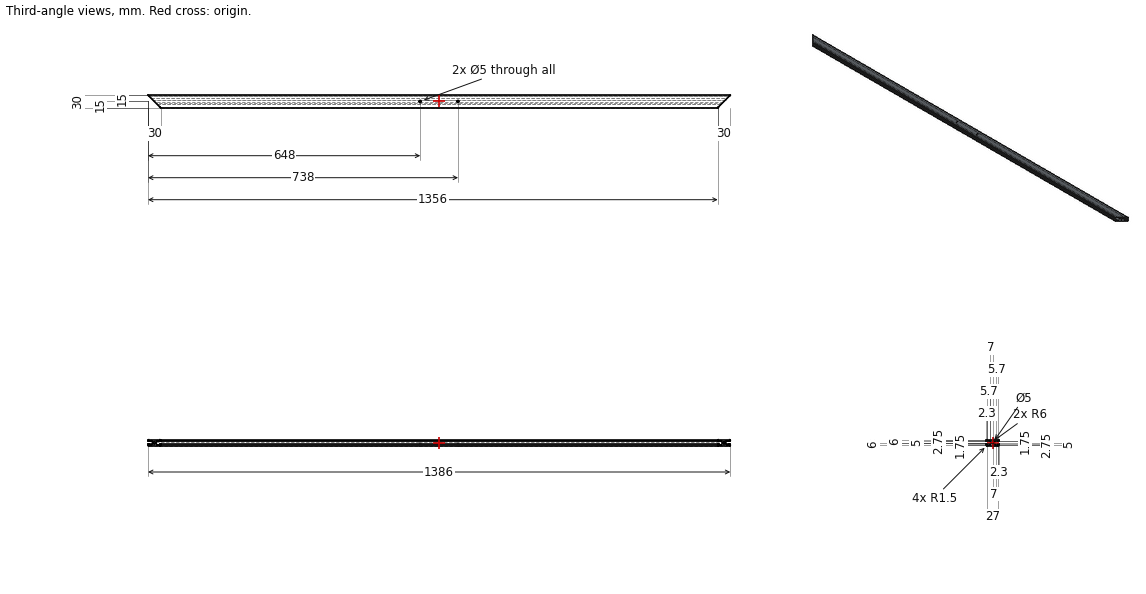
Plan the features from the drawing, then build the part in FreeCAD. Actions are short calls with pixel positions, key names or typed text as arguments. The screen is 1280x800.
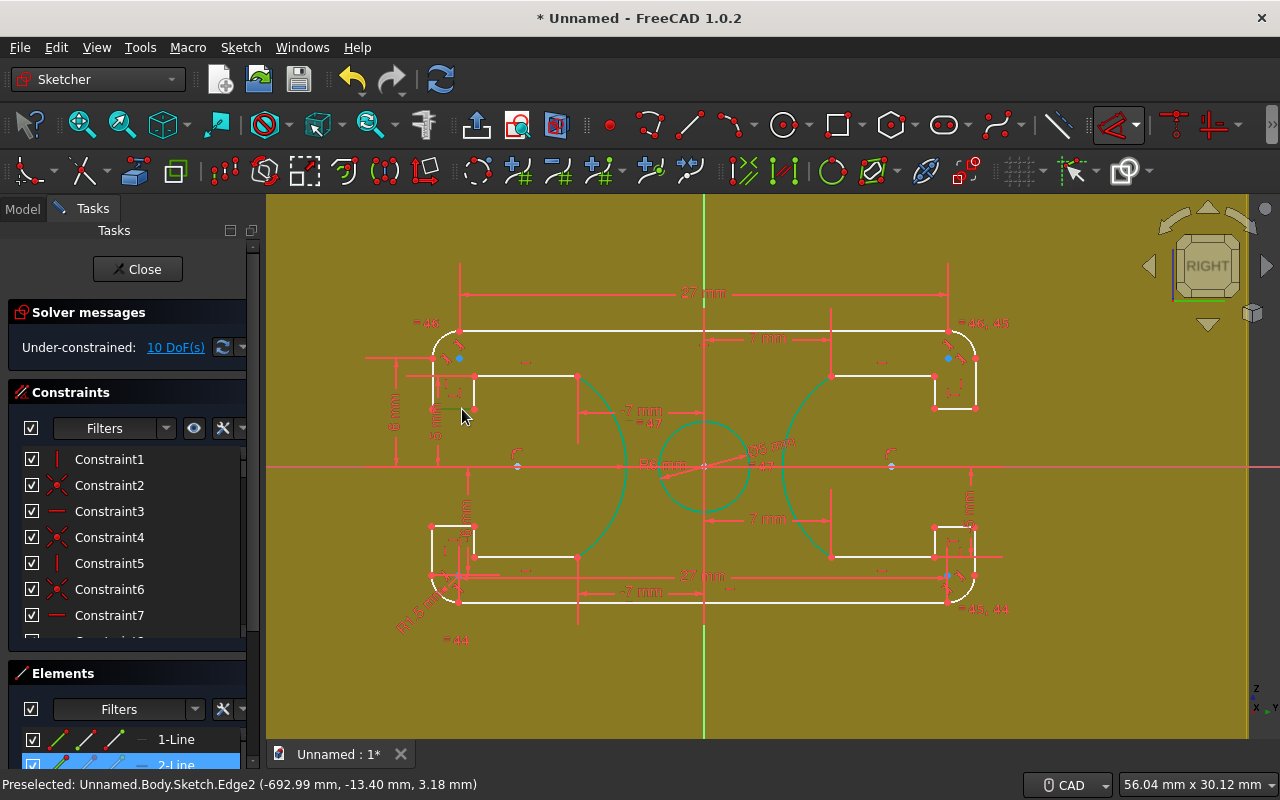
click(1138, 126)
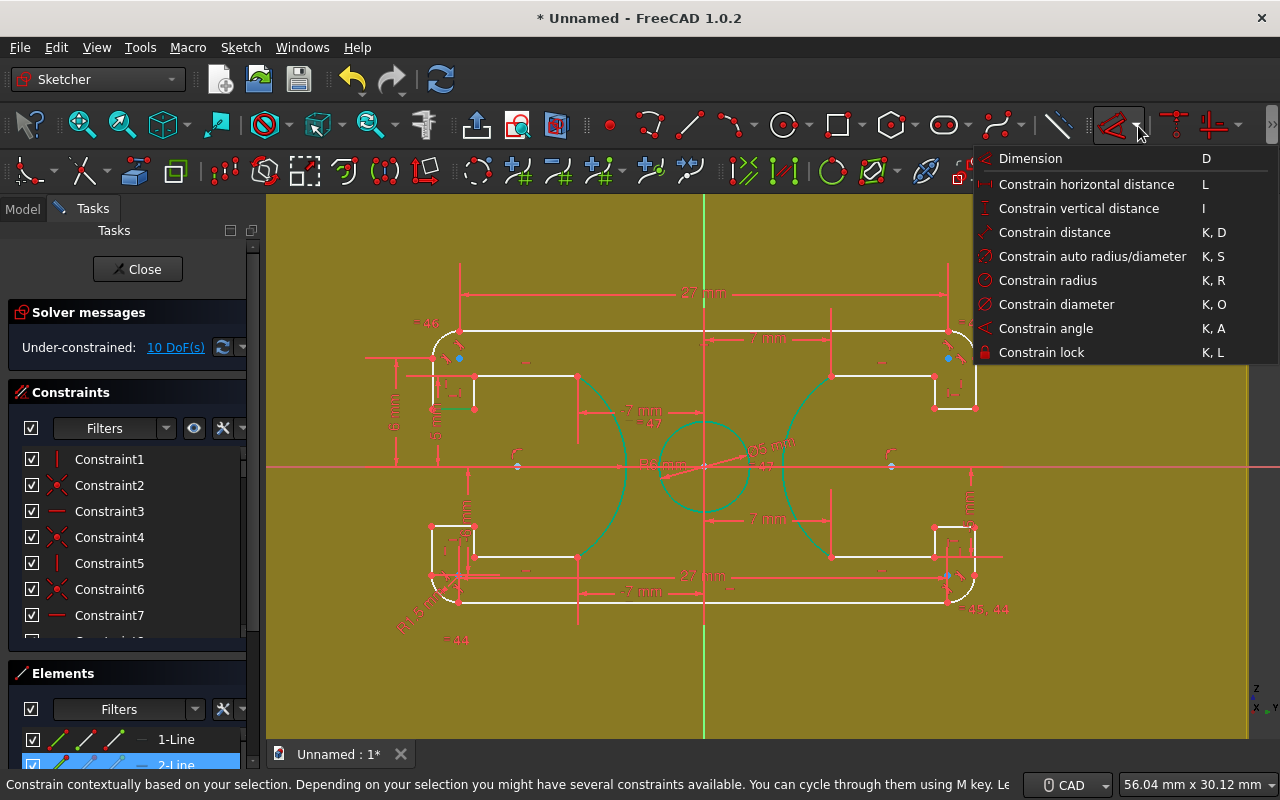
click(1126, 184)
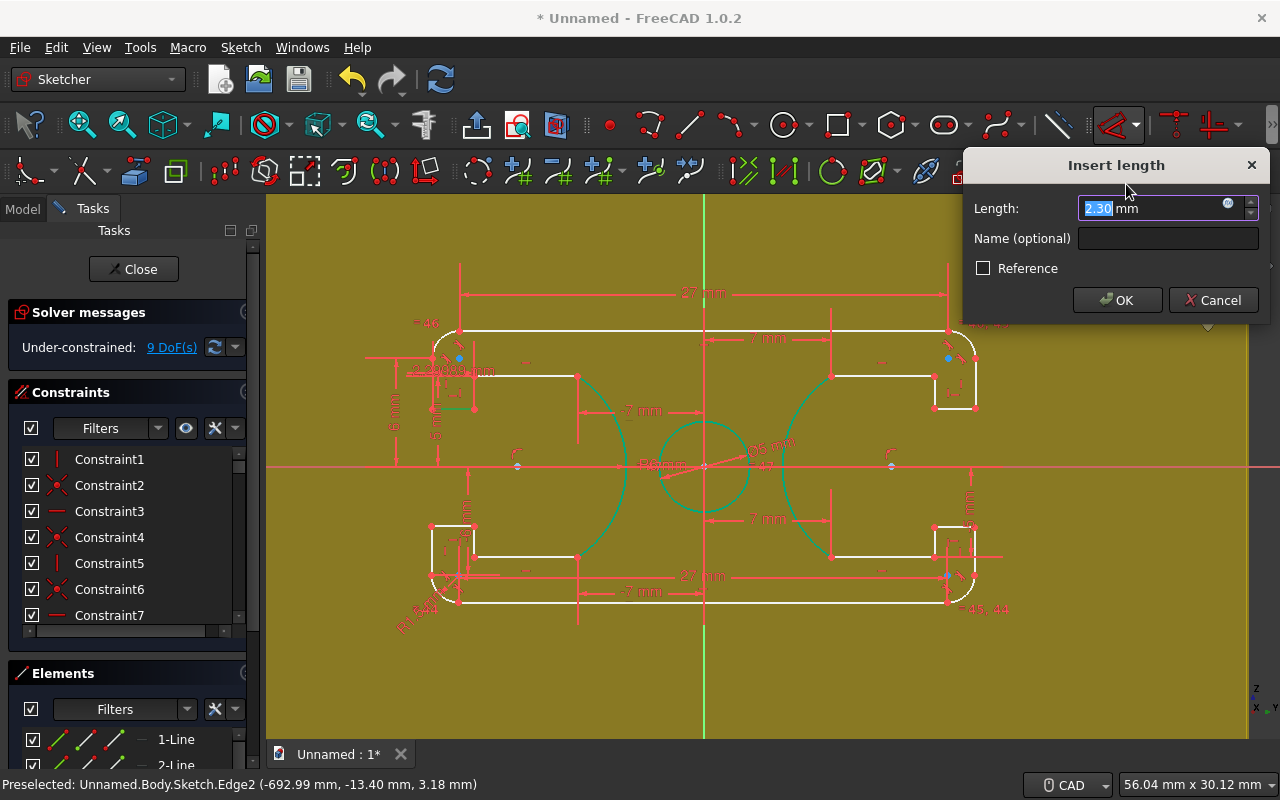
text(2.3)
key(Return)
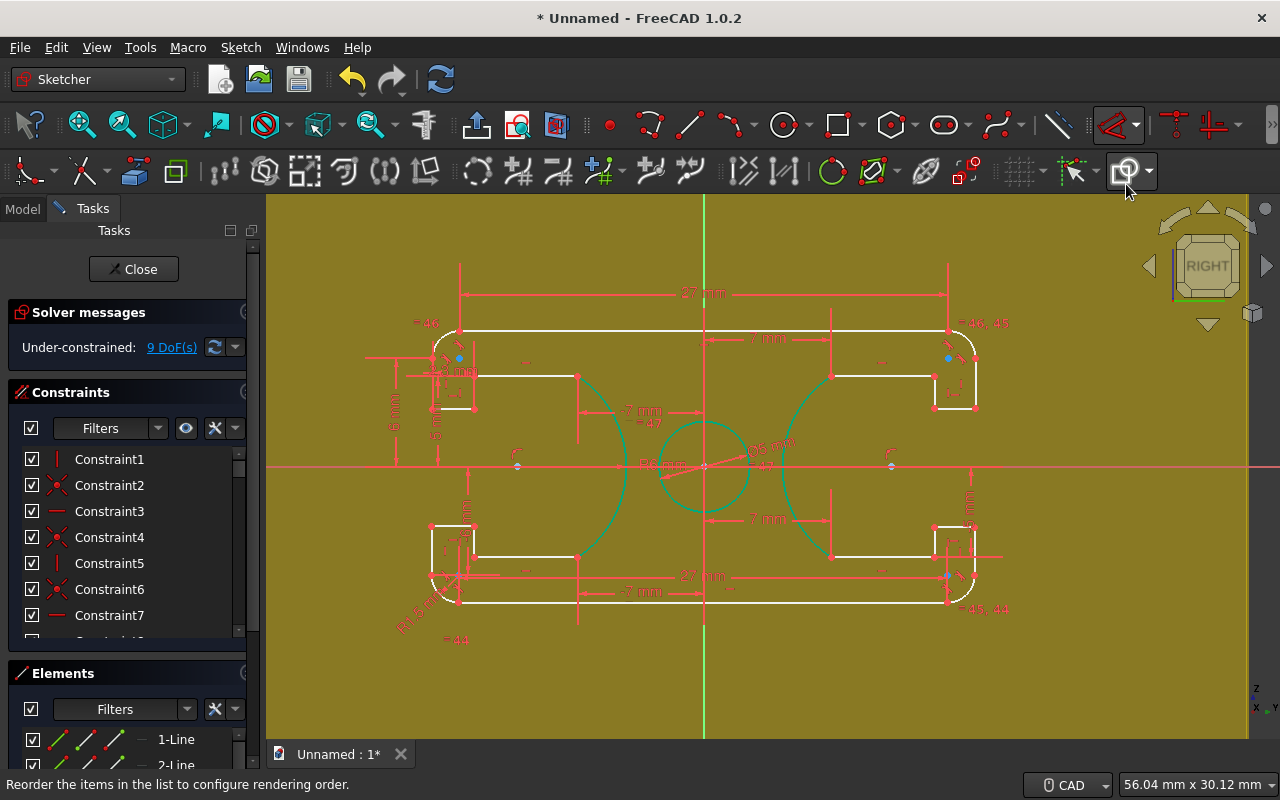
click(505, 376)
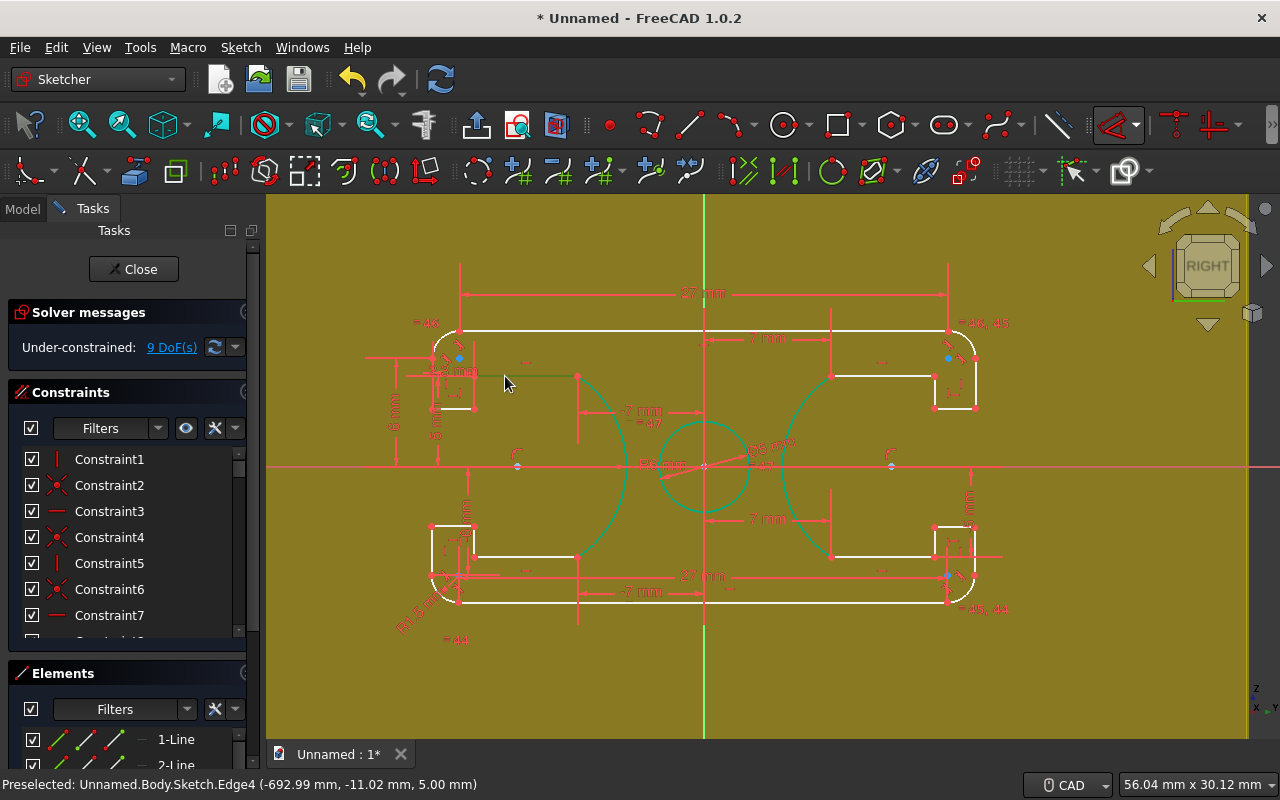
click(1138, 126)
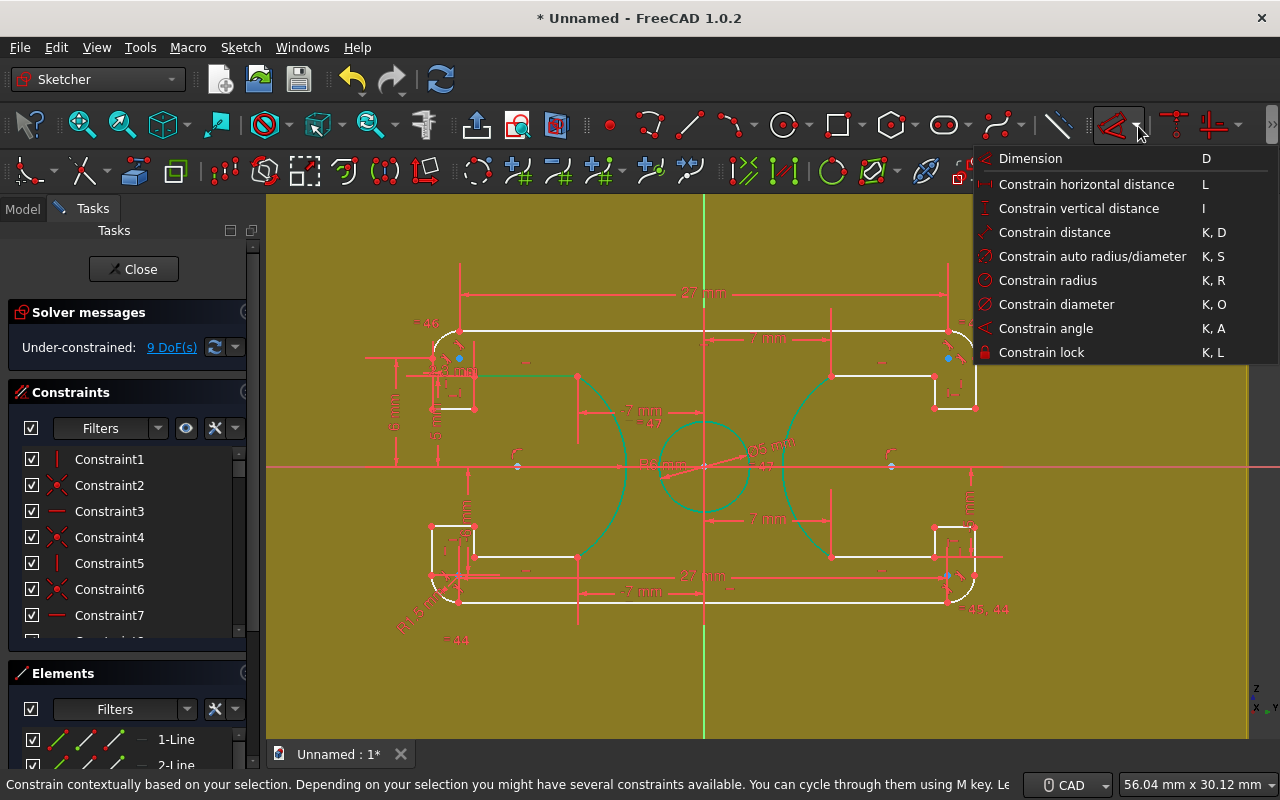
click(1126, 184)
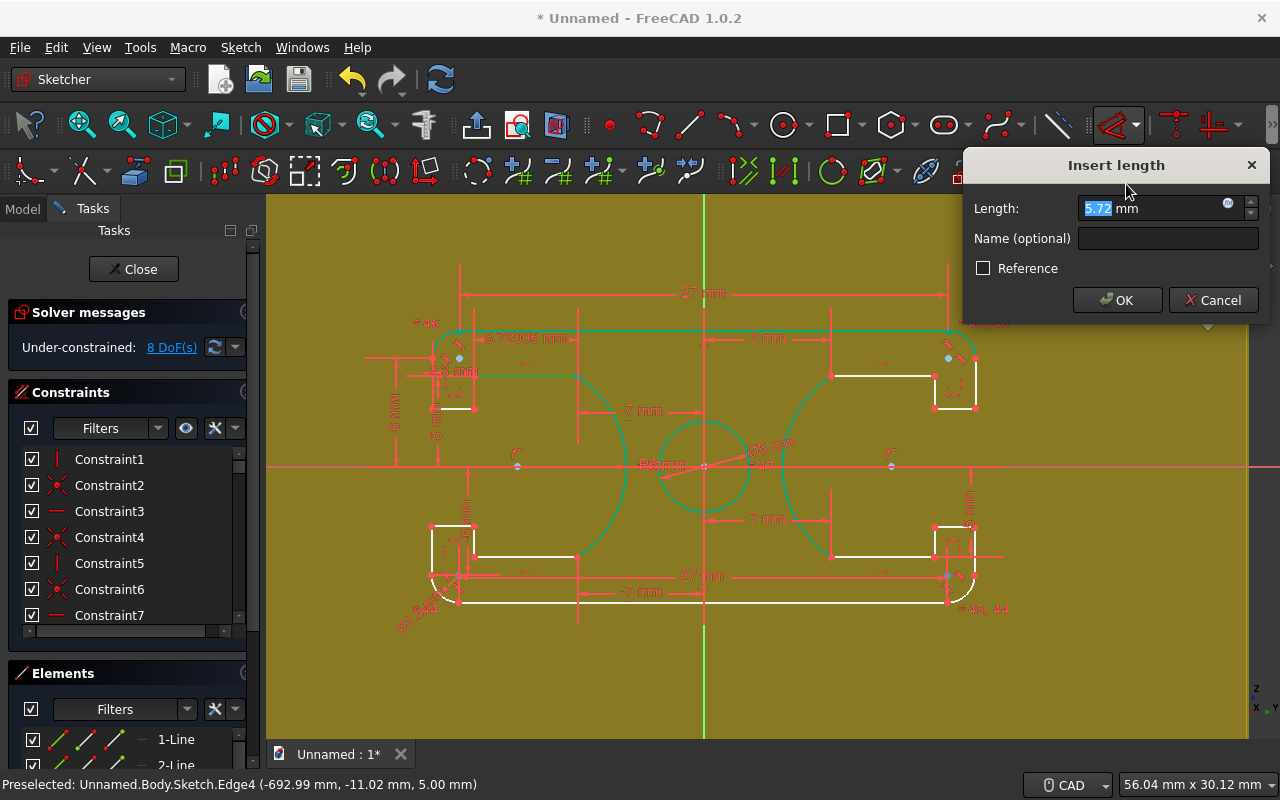
text(5.7)
key(Return)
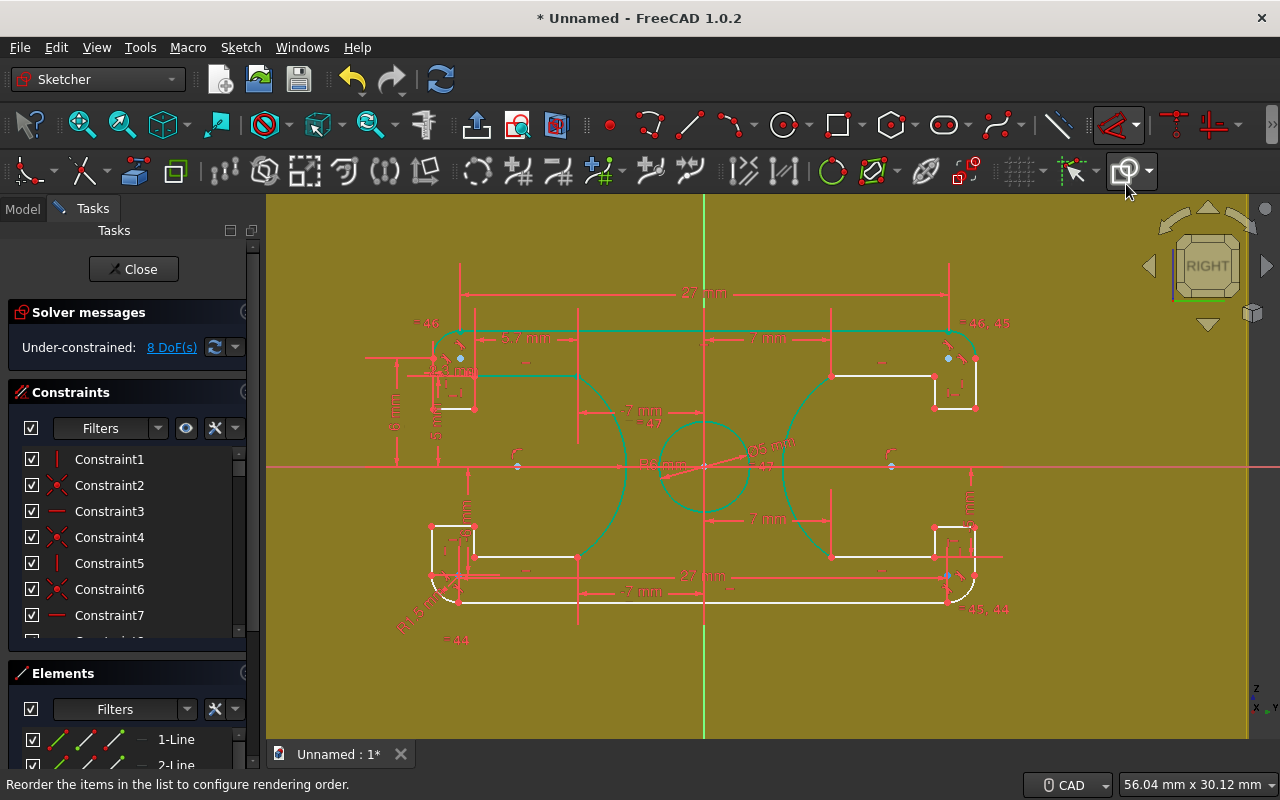
click(547, 557)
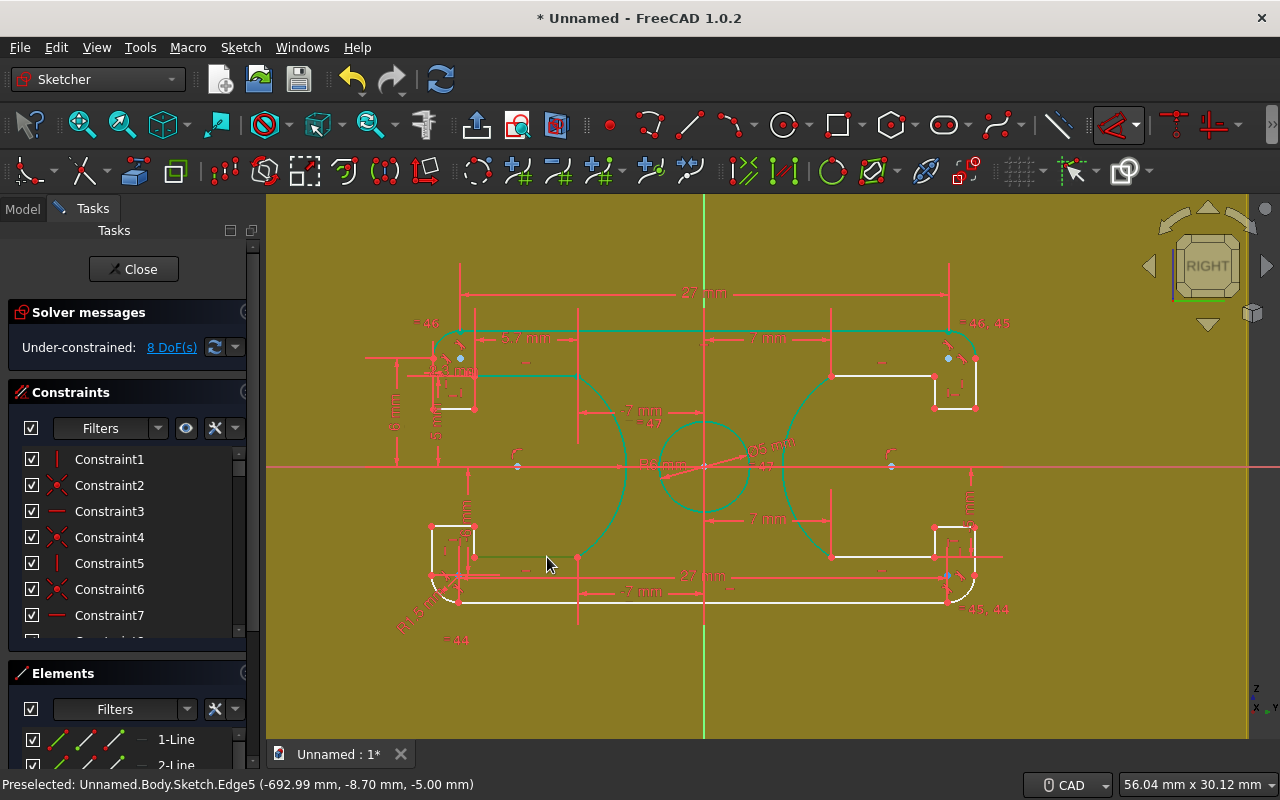
click(1138, 126)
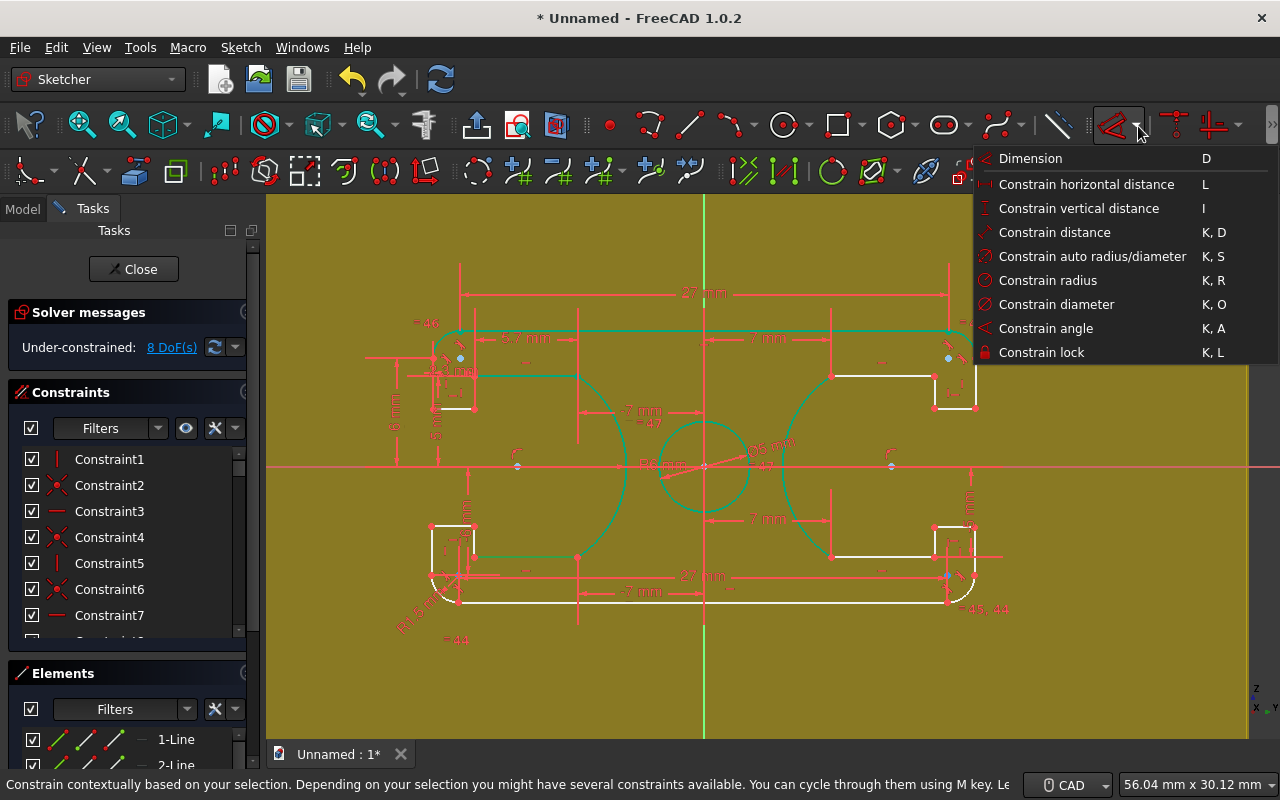
click(1126, 184)